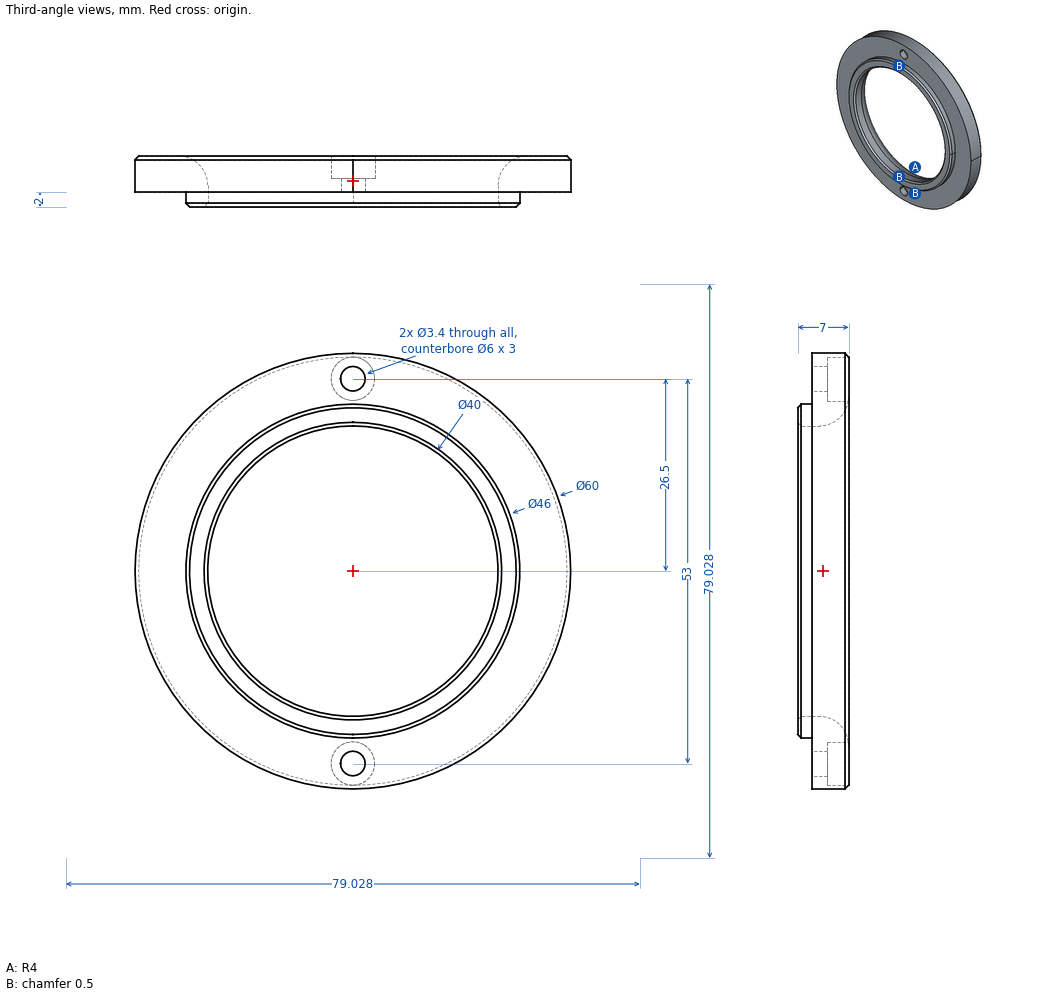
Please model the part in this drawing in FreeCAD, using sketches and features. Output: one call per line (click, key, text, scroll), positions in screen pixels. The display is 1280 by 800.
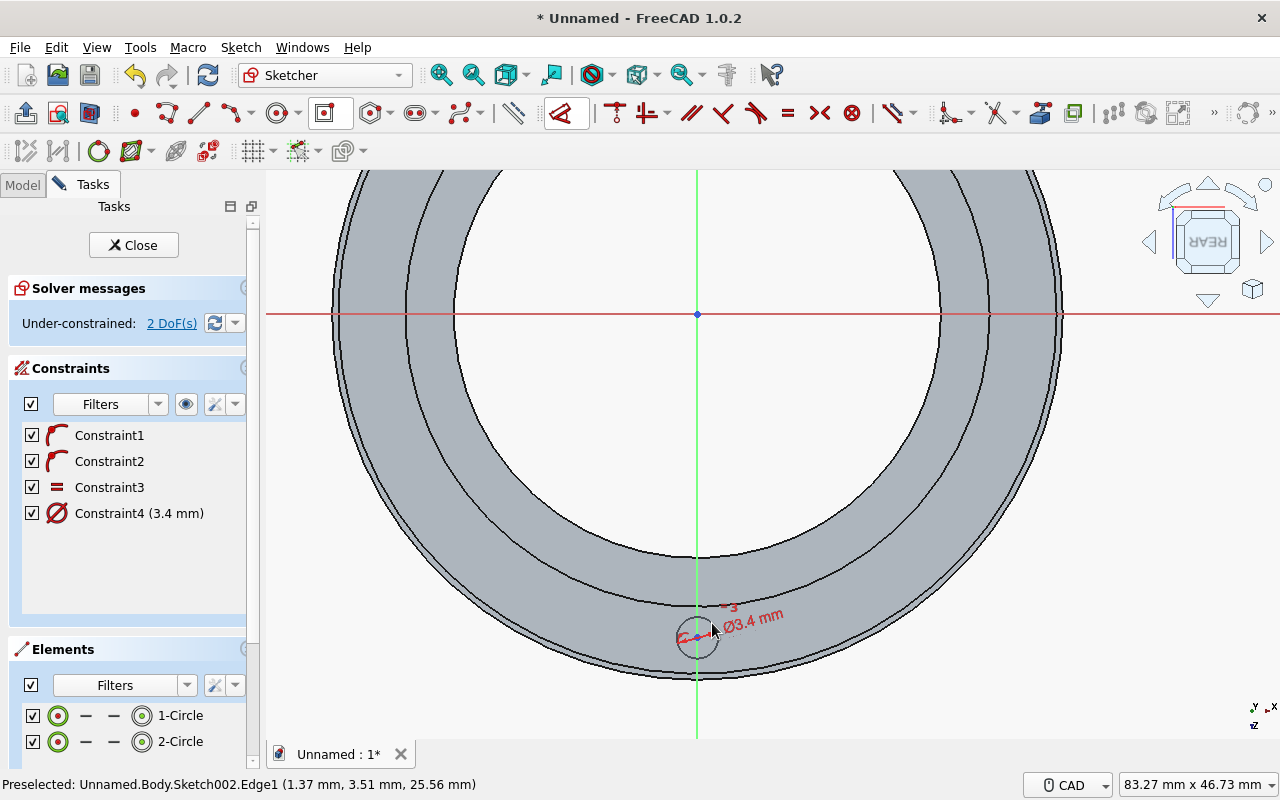
click(697, 638)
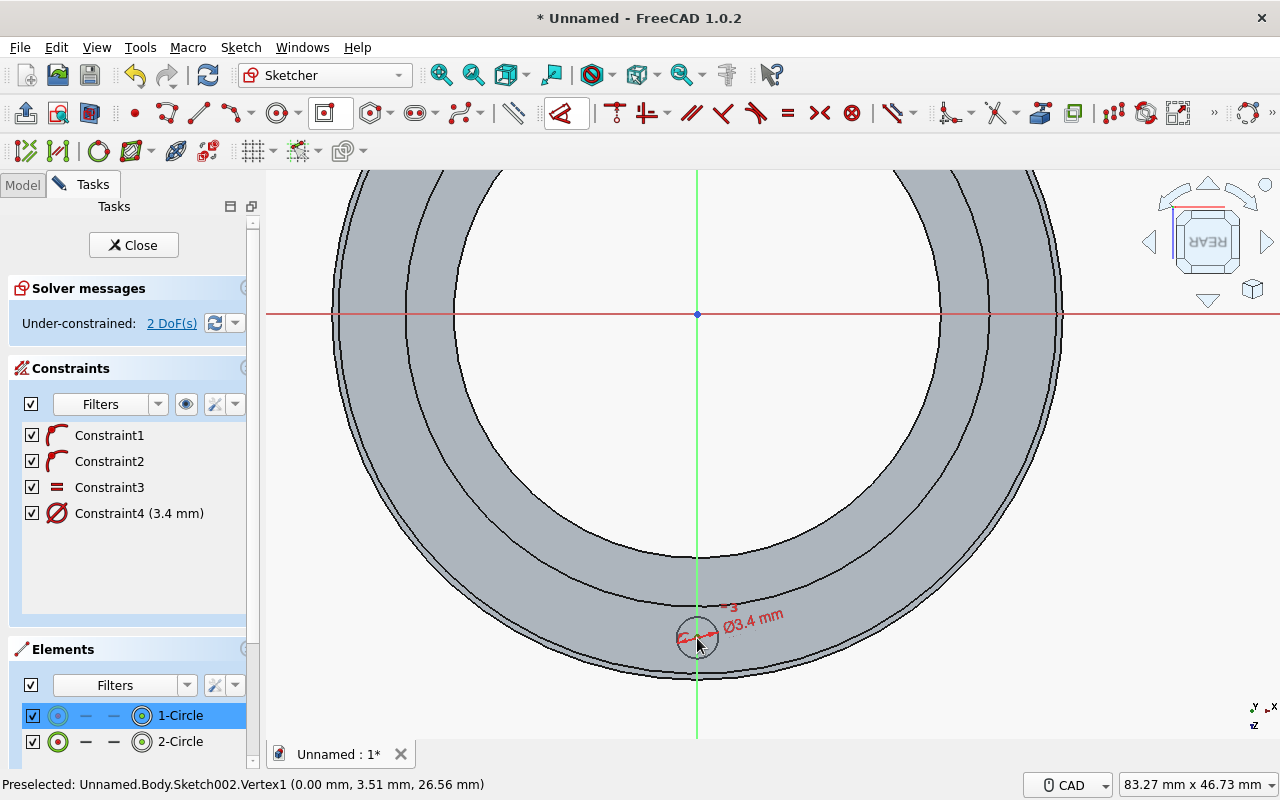
scroll(713, 625, down, 3)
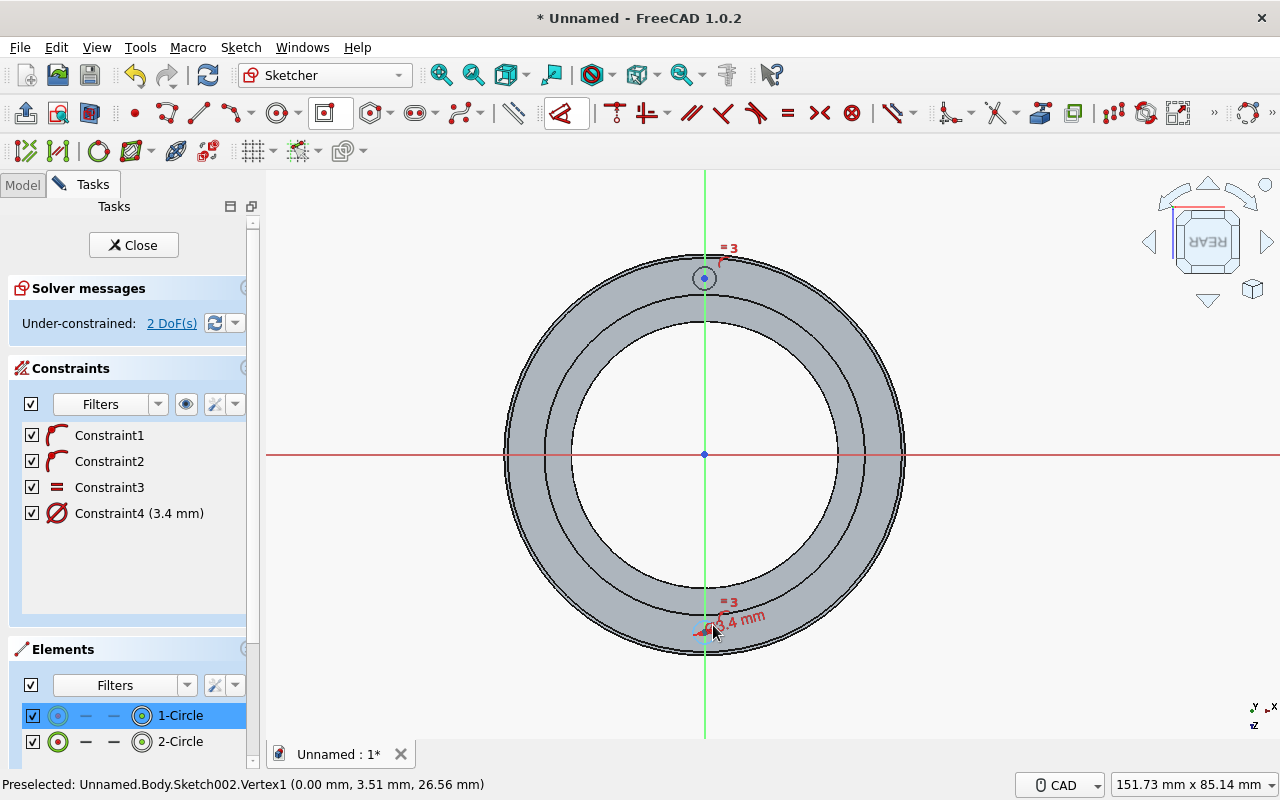
click(705, 278)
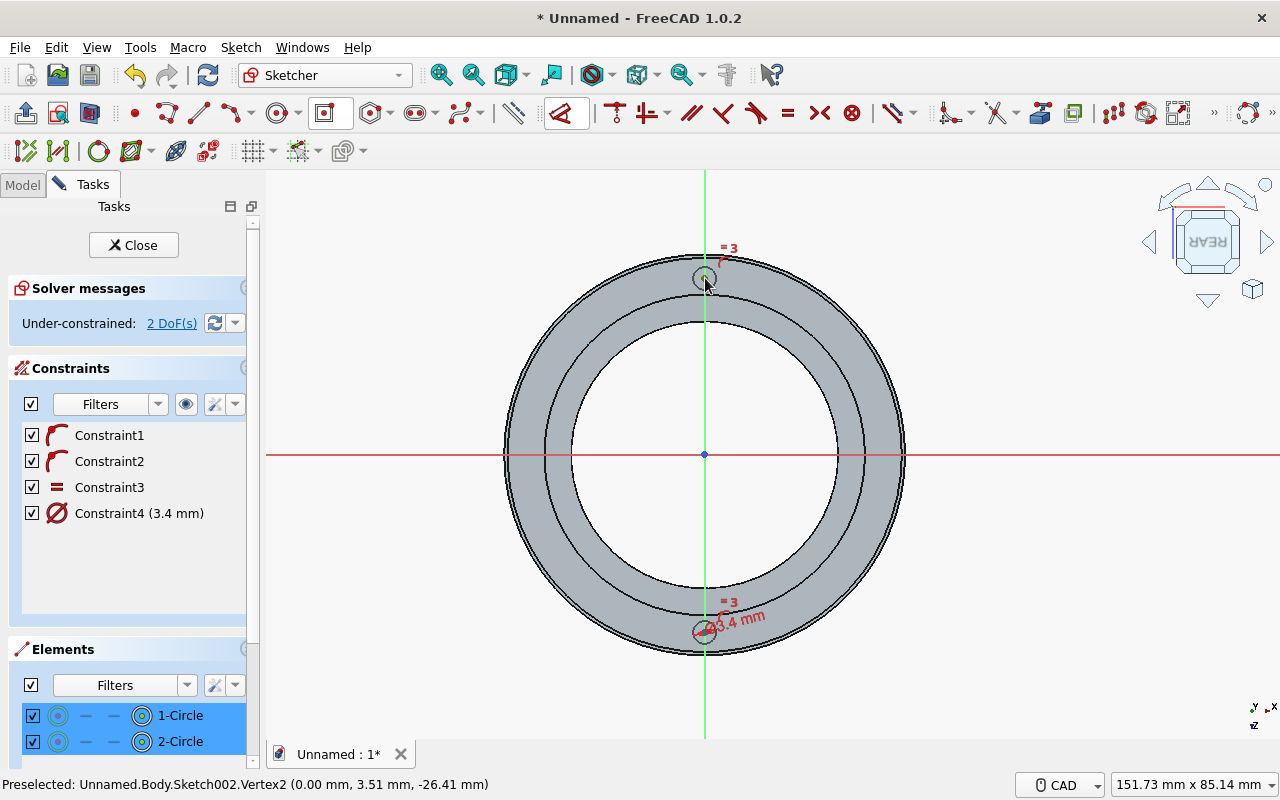
click(584, 114)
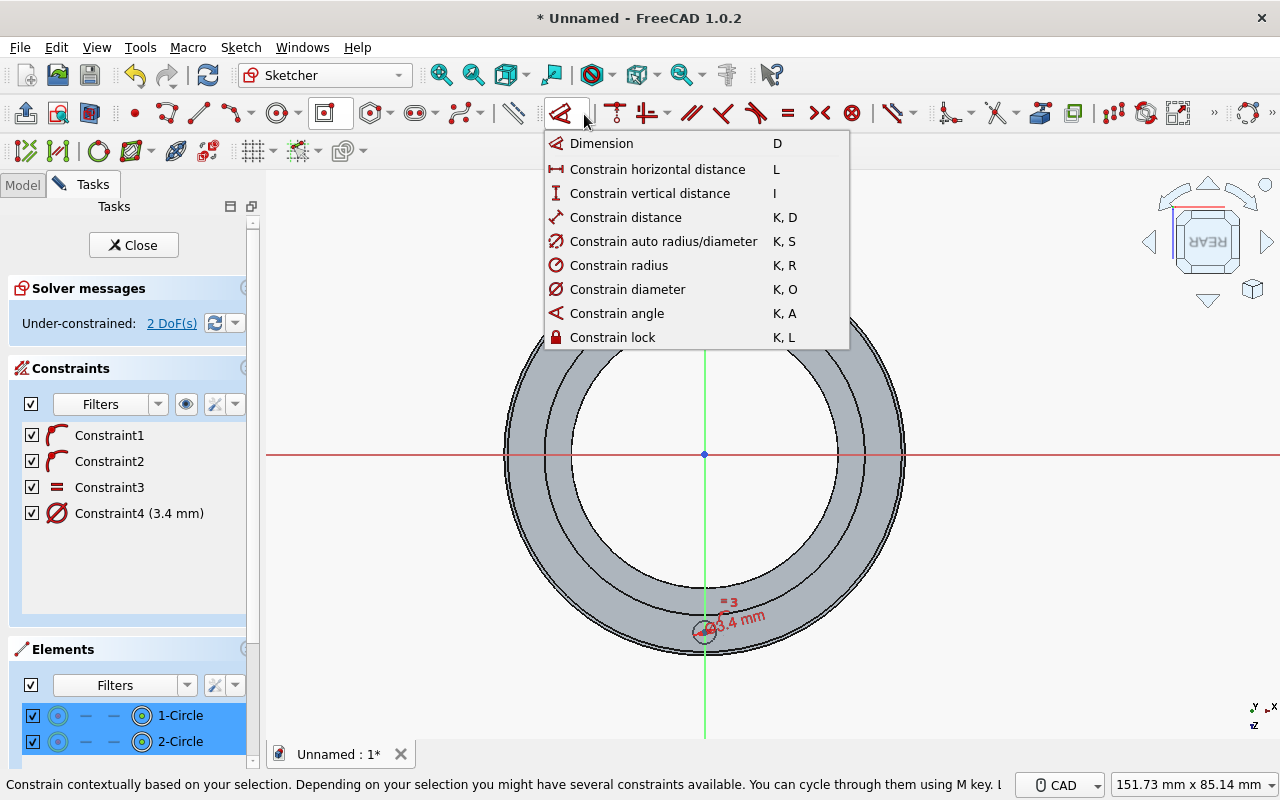
click(697, 193)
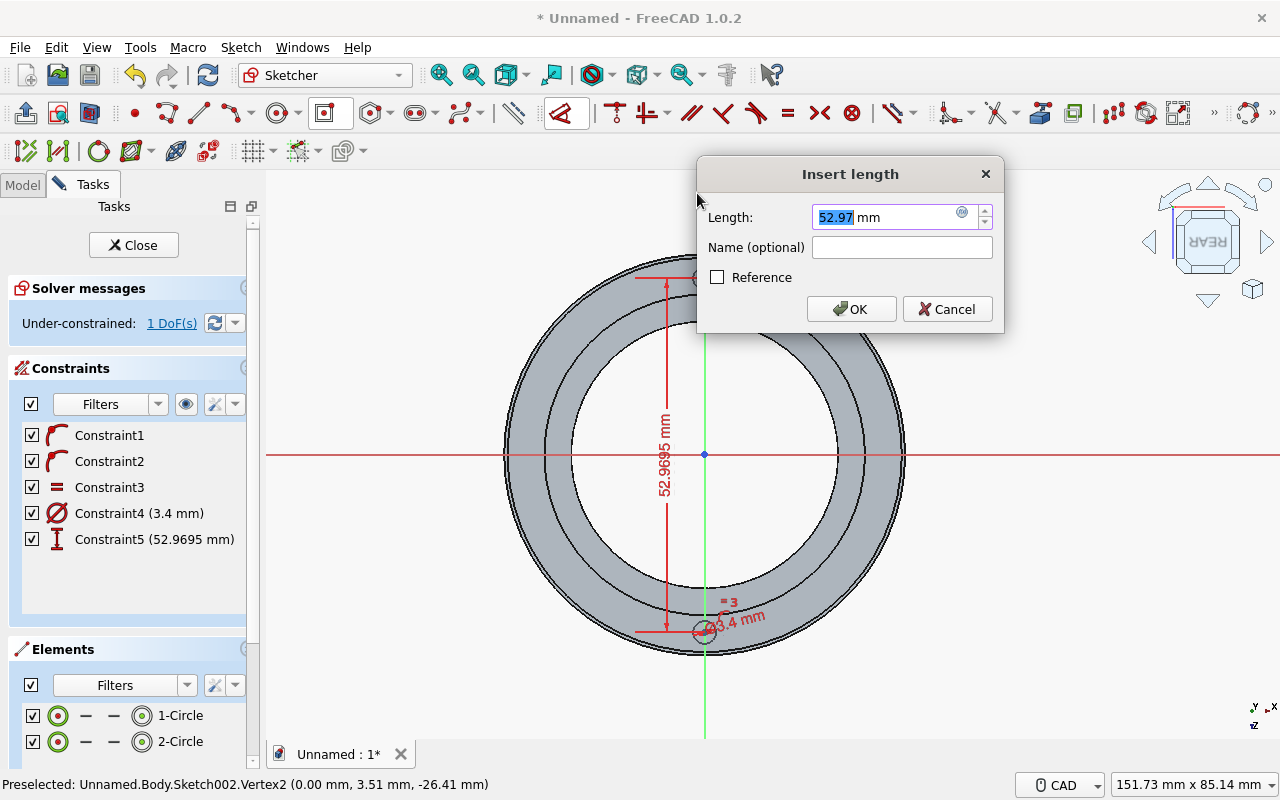
text(53)
key(Return)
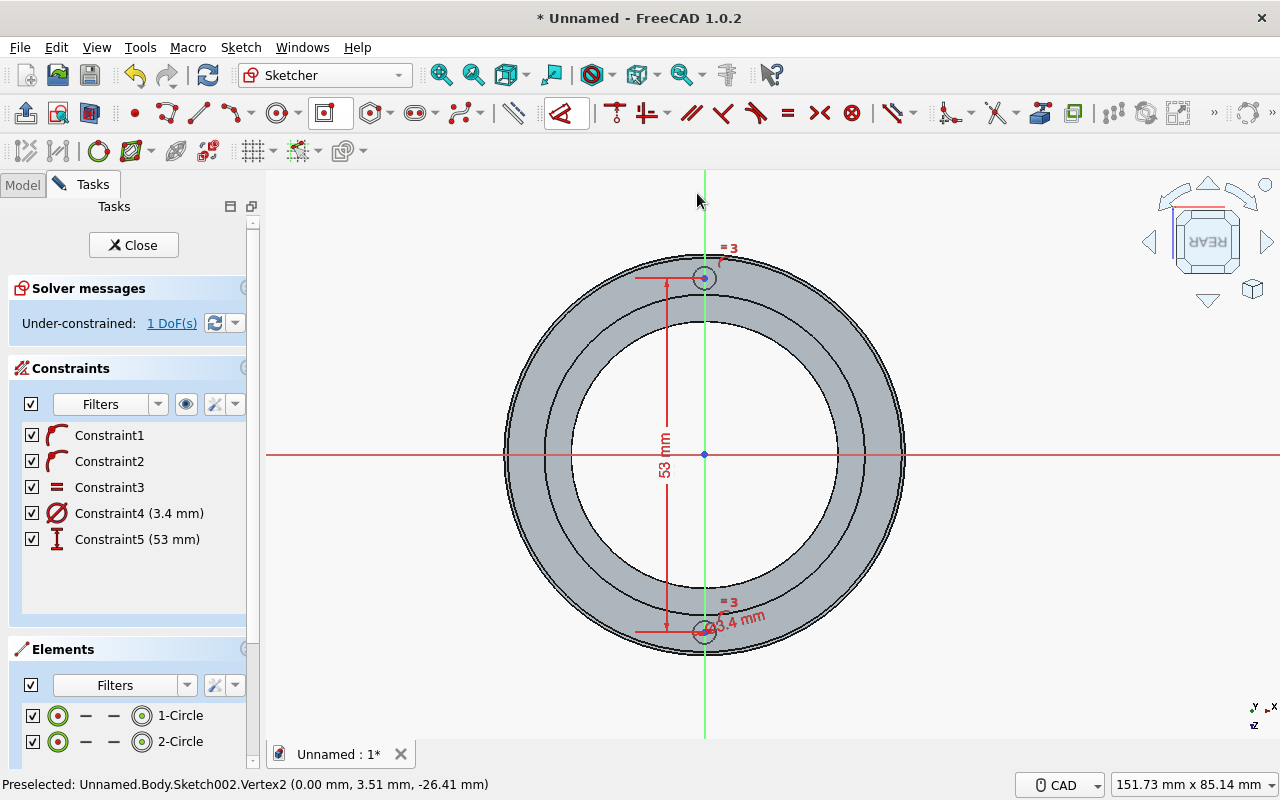
click(705, 632)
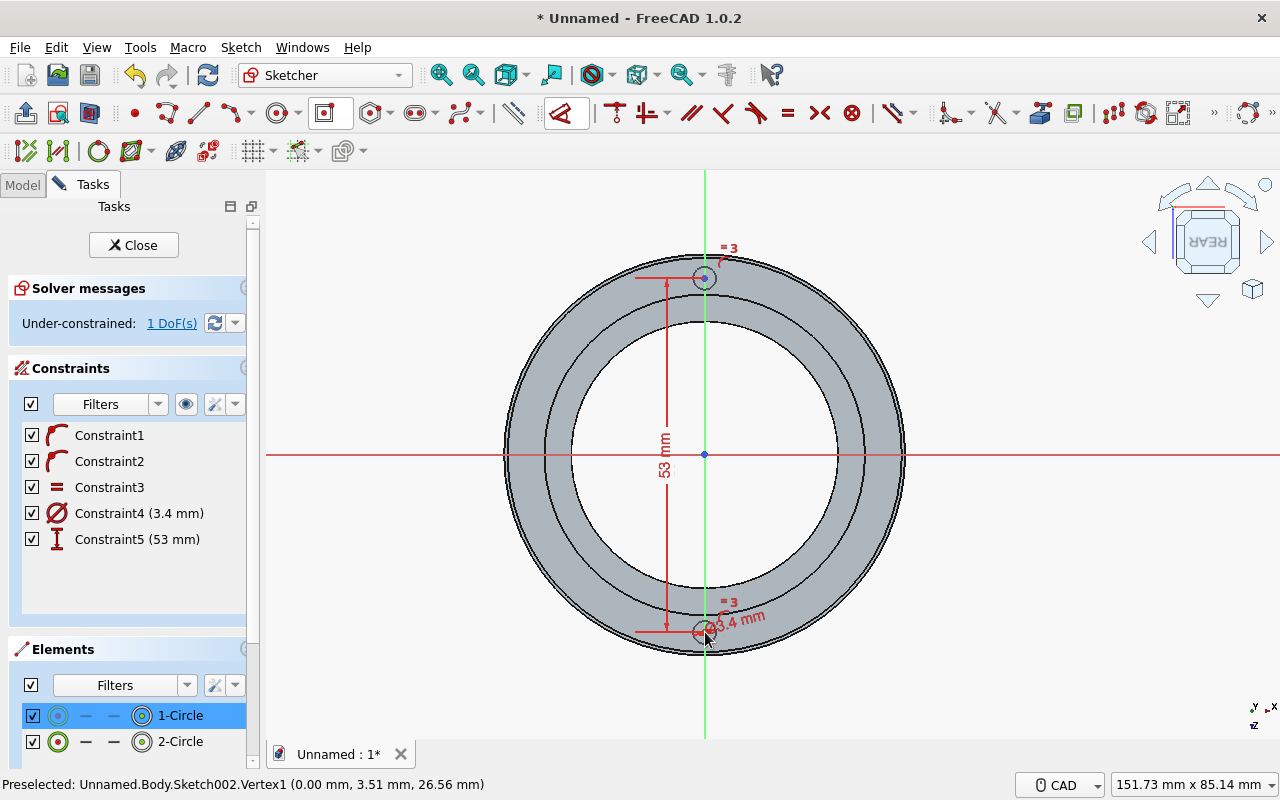
click(584, 114)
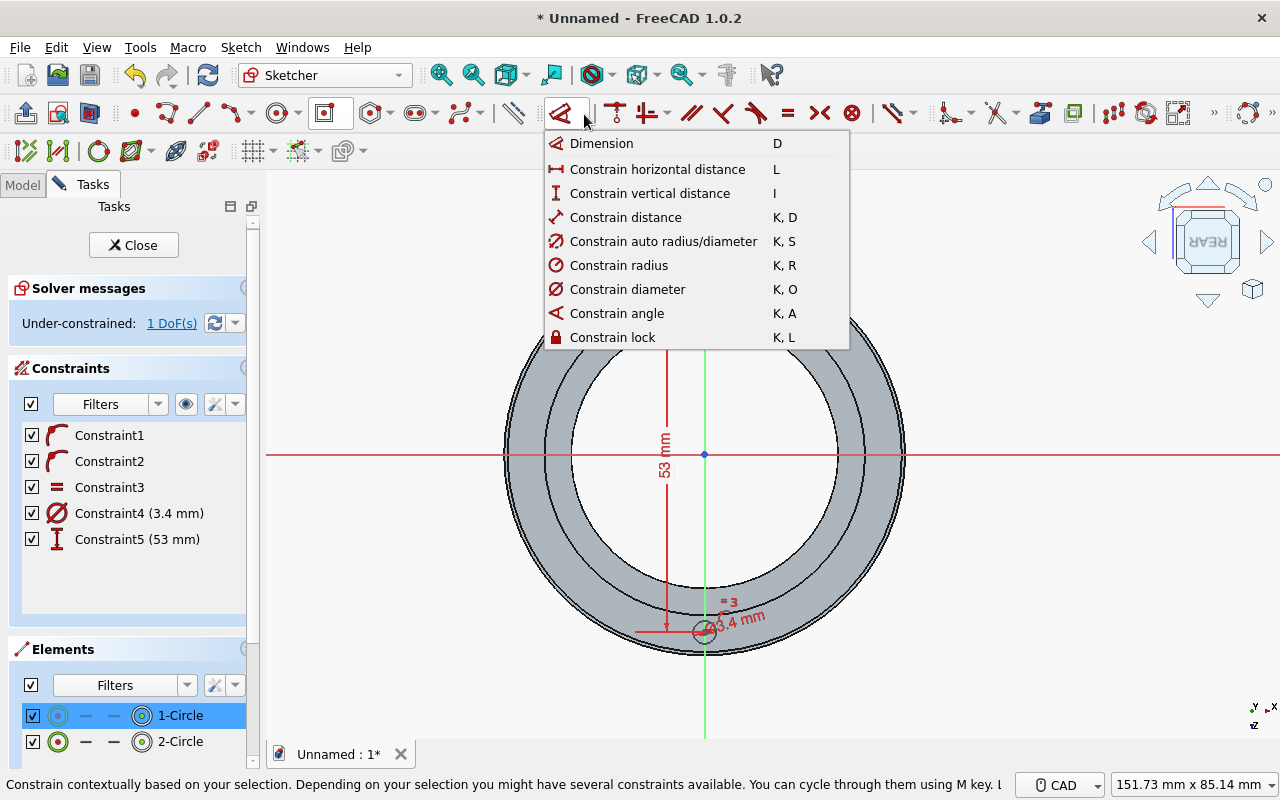
click(697, 193)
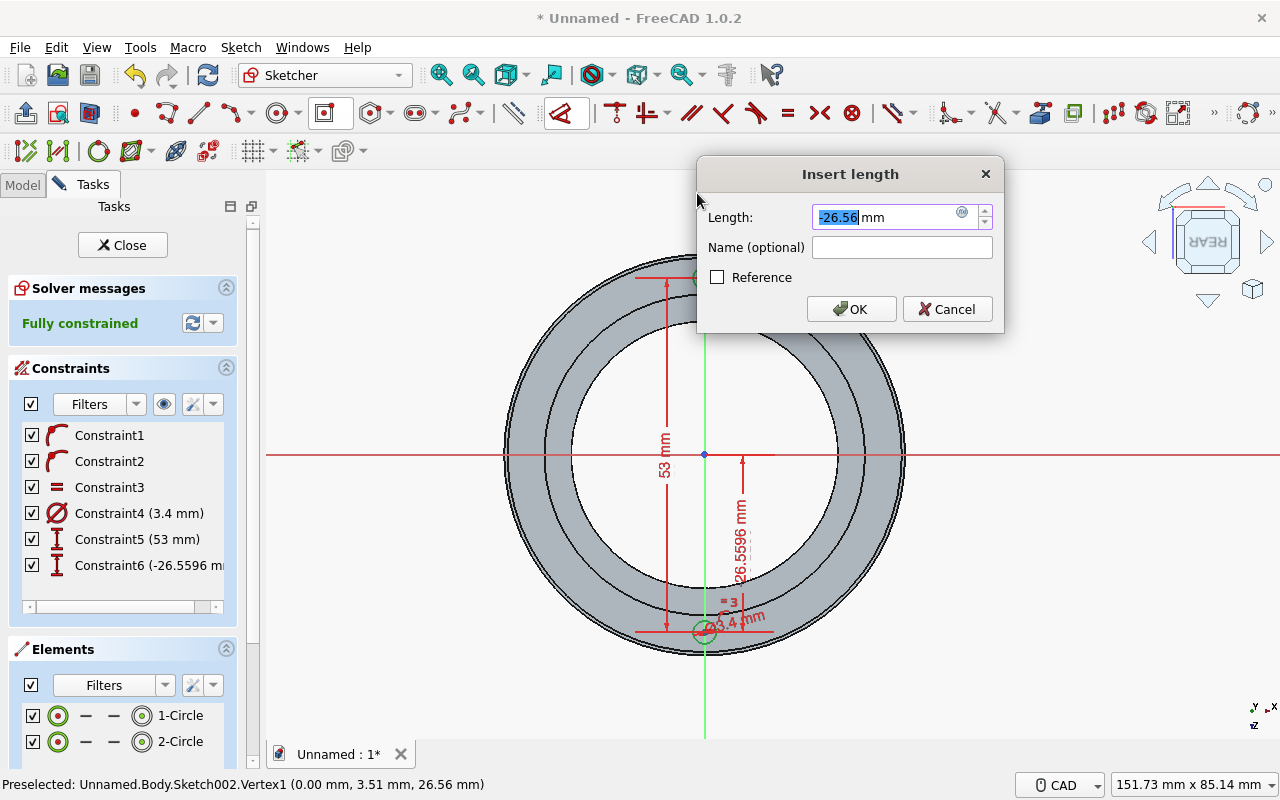
text(-26.5)
key(Return)